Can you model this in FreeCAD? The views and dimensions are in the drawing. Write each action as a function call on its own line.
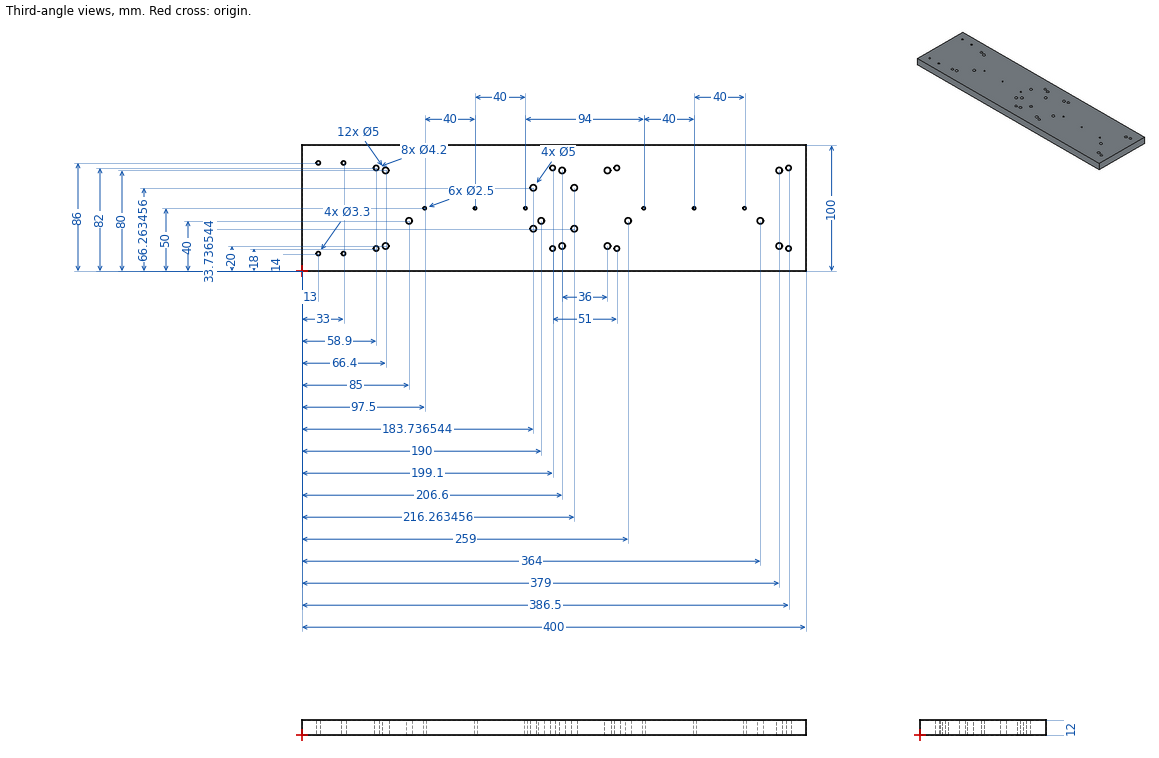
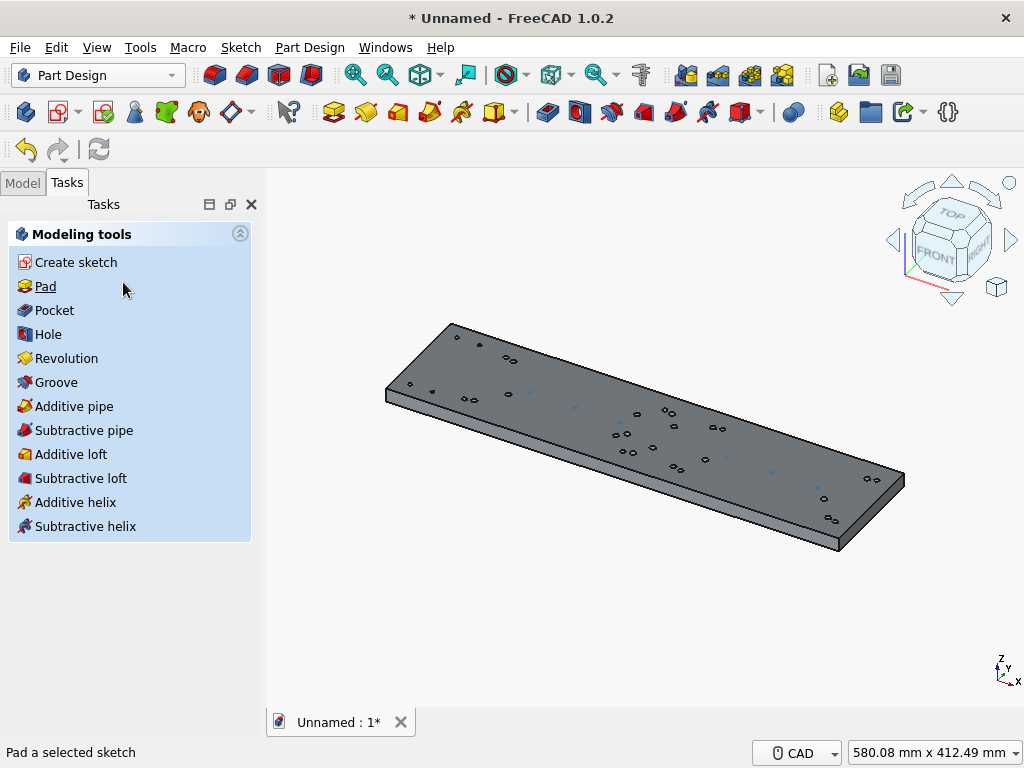
click(548, 112)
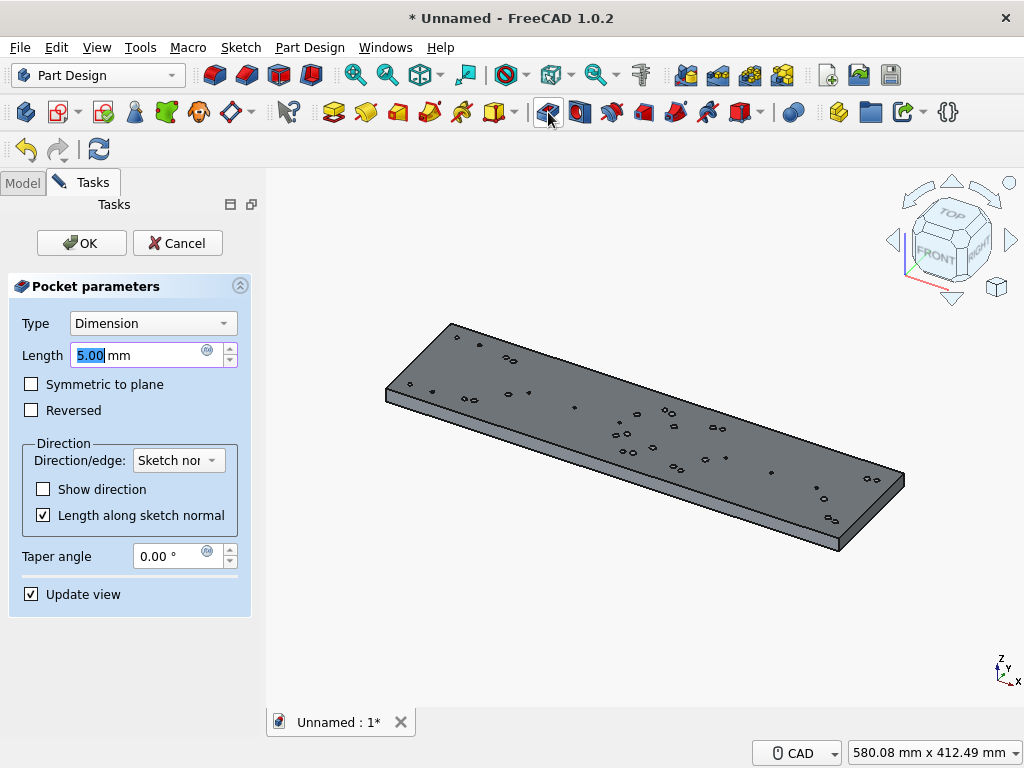
click(212, 324)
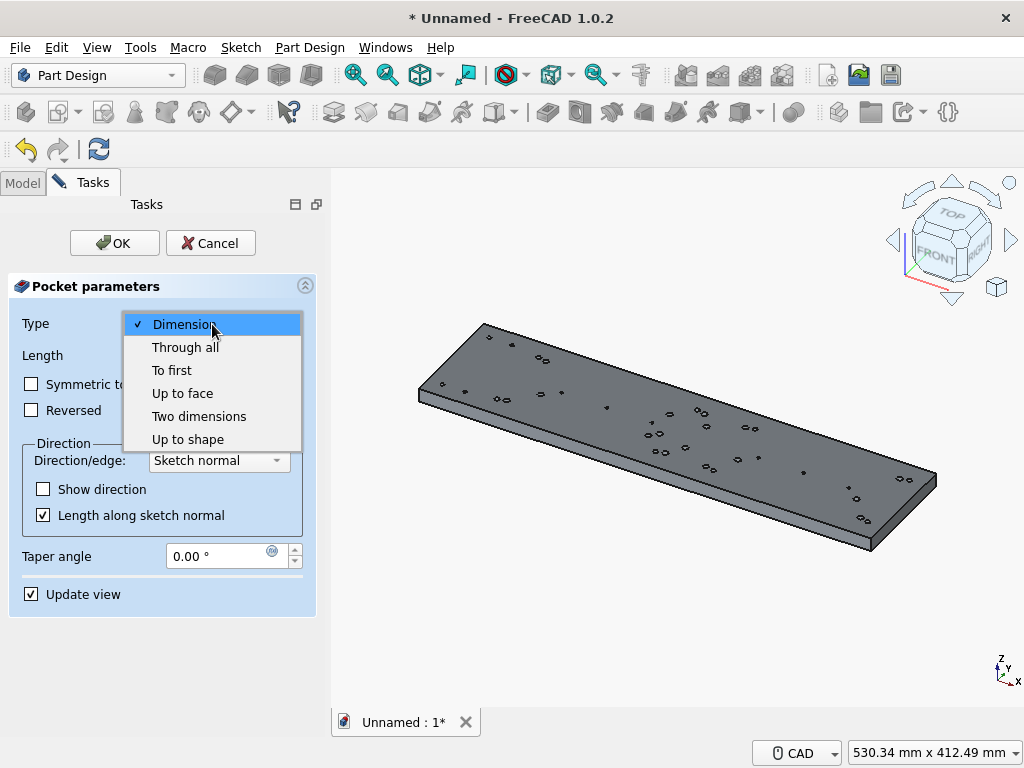
click(212, 348)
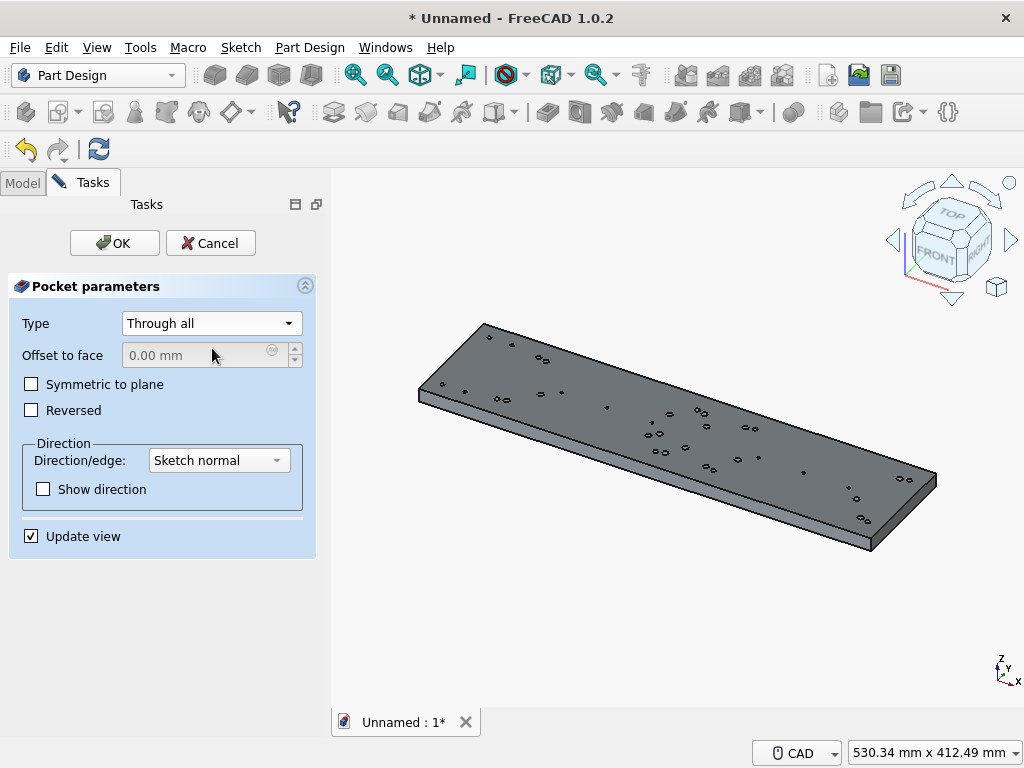
click(115, 243)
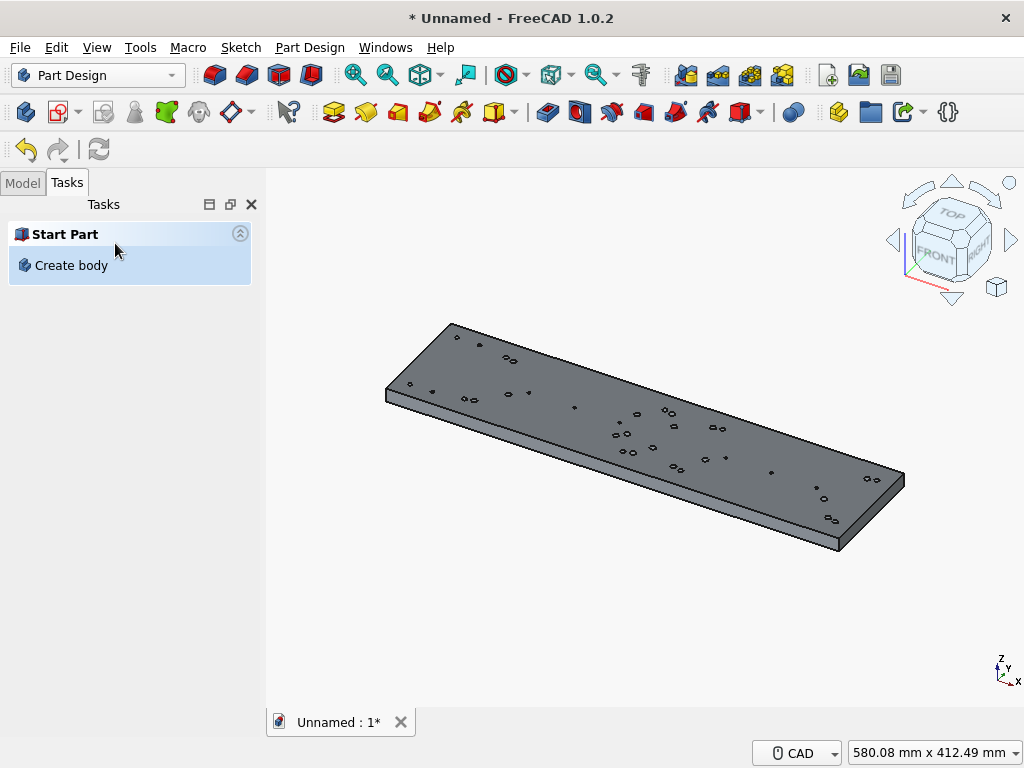
key(0)